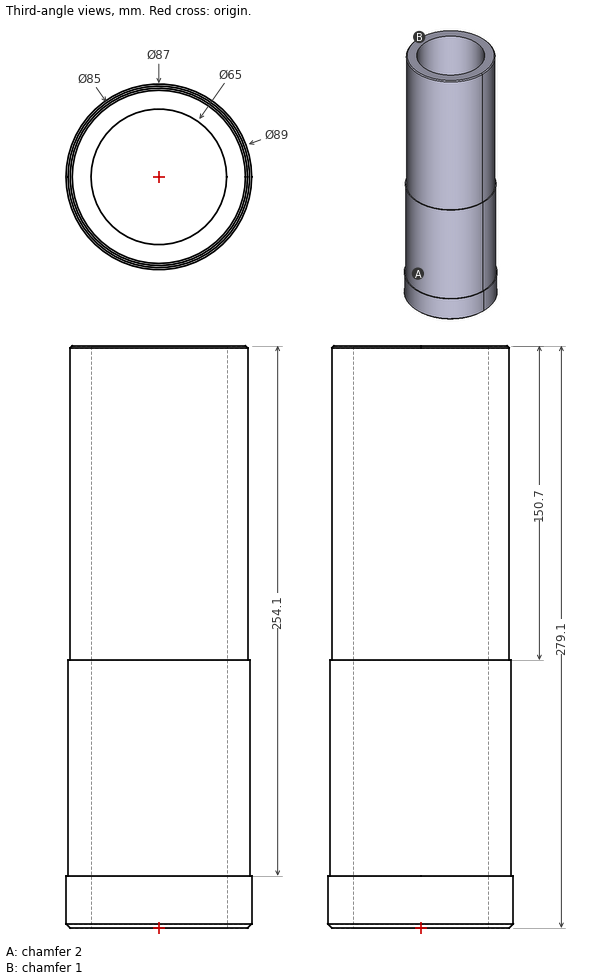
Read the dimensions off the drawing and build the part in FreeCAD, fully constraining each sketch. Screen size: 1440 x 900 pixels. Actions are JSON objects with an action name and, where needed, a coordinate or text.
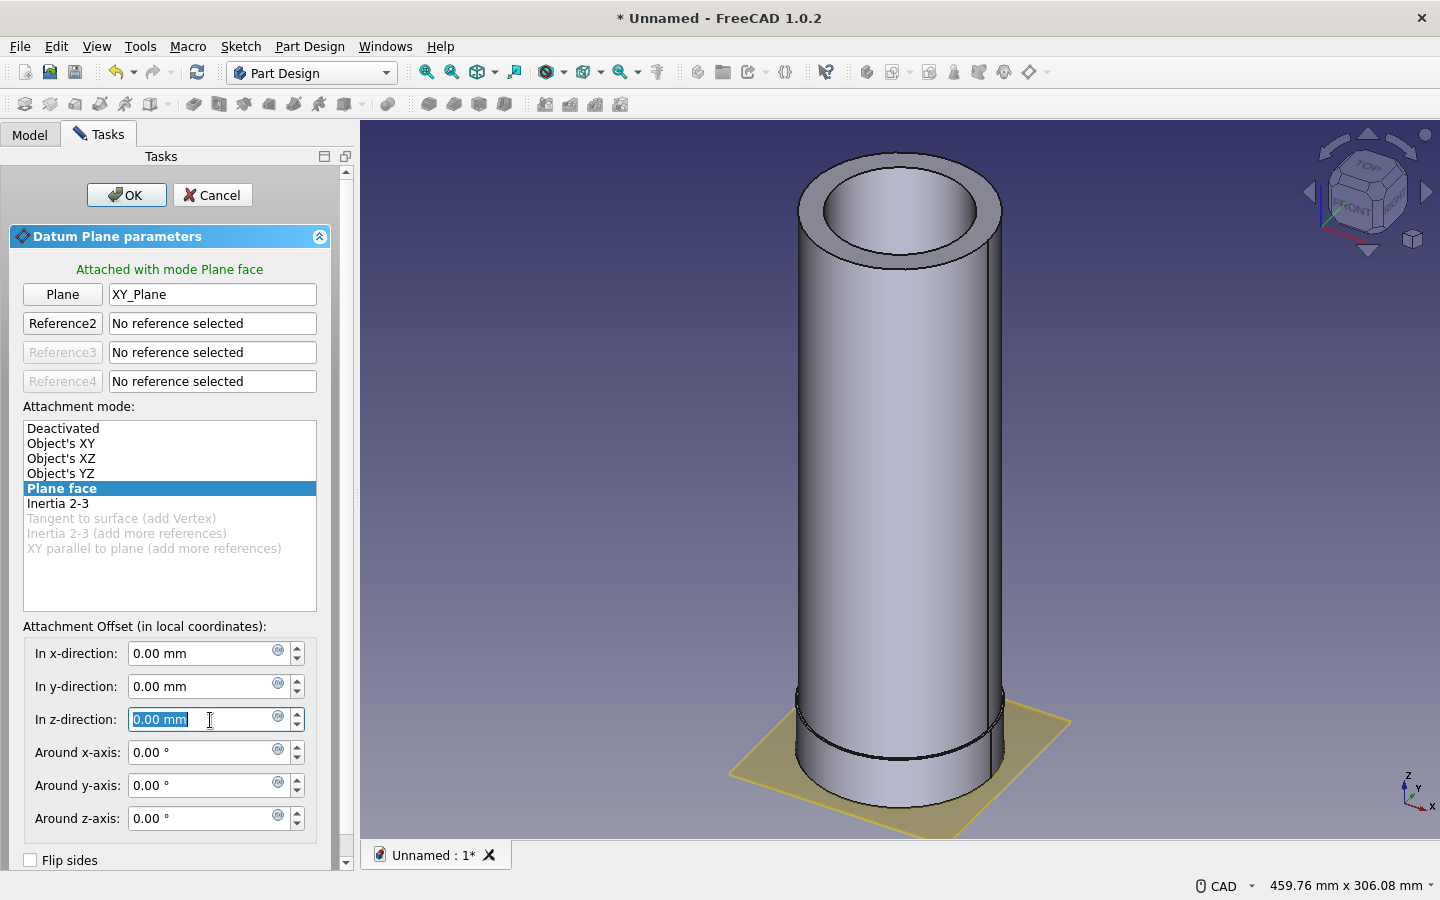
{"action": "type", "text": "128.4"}
{"action": "key", "text": "Tab"}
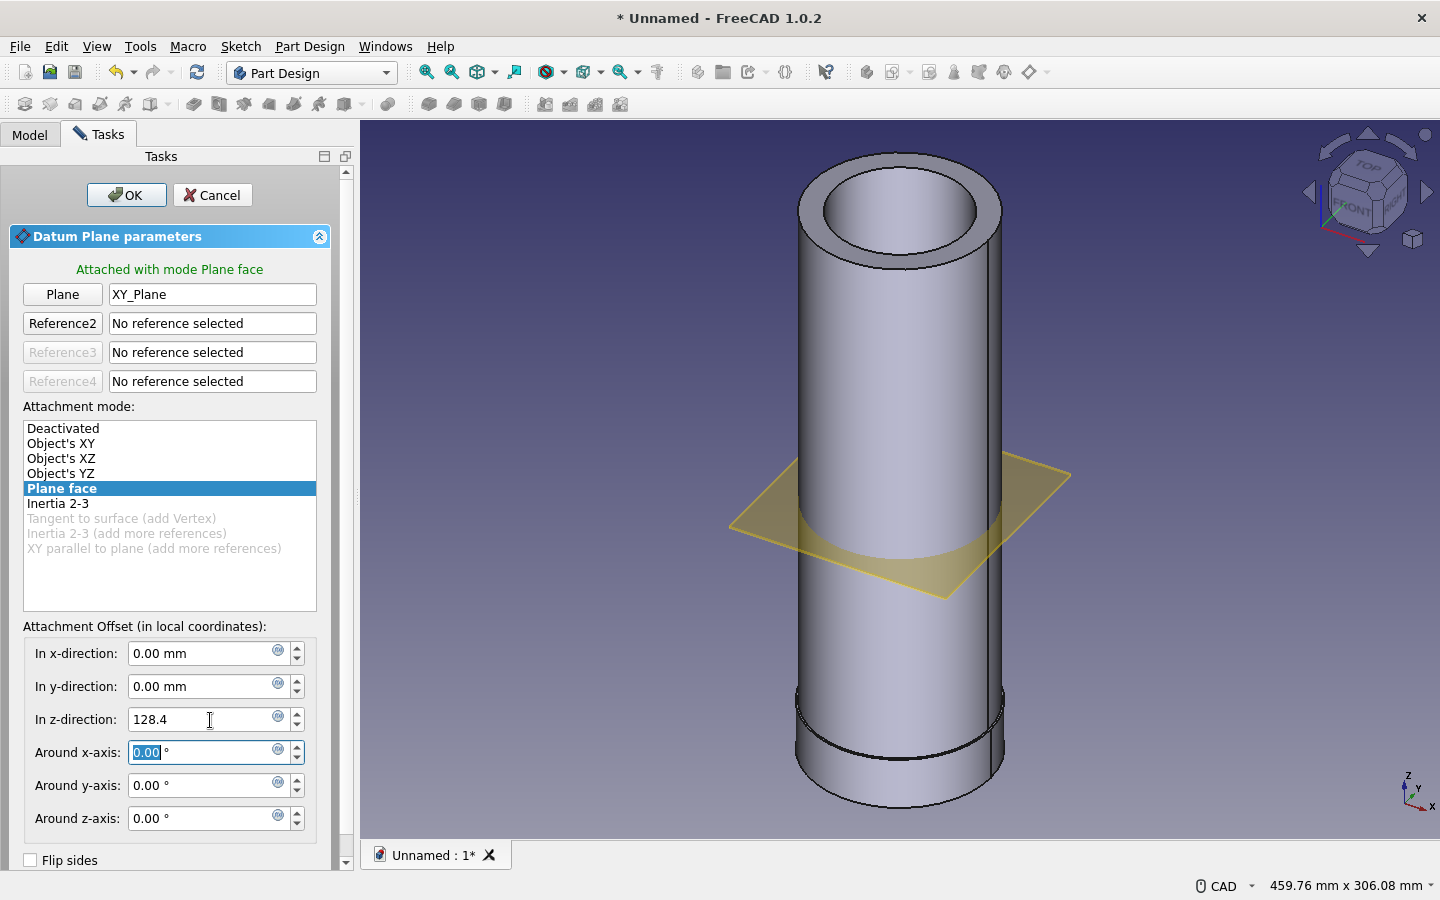
{"action": "left_click", "coordinate": [127, 195]}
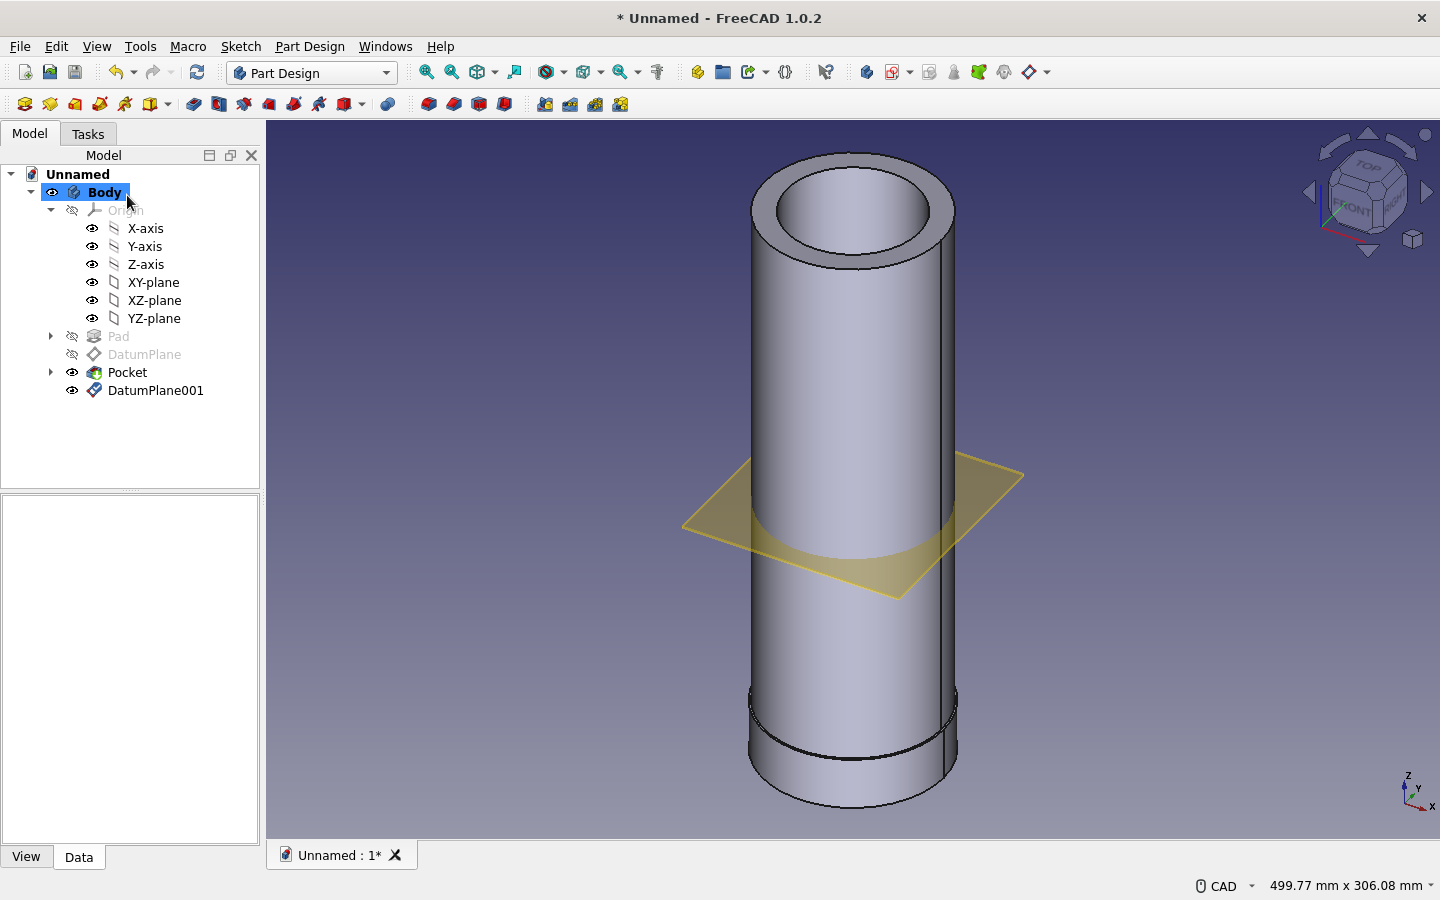
{"action": "left_click", "coordinate": [117, 390]}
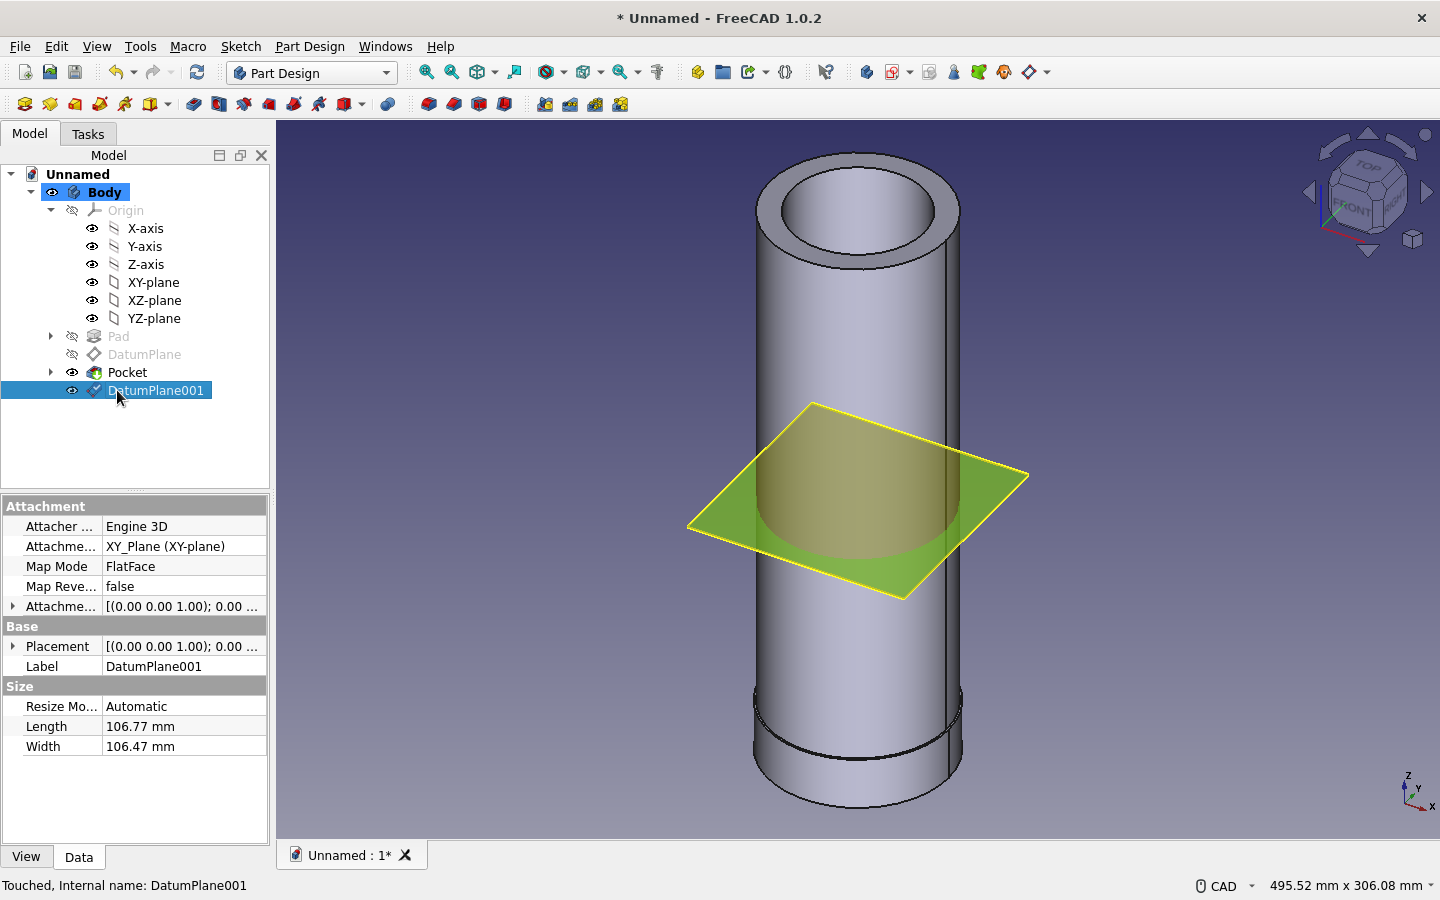
{"action": "left_click", "coordinate": [892, 72]}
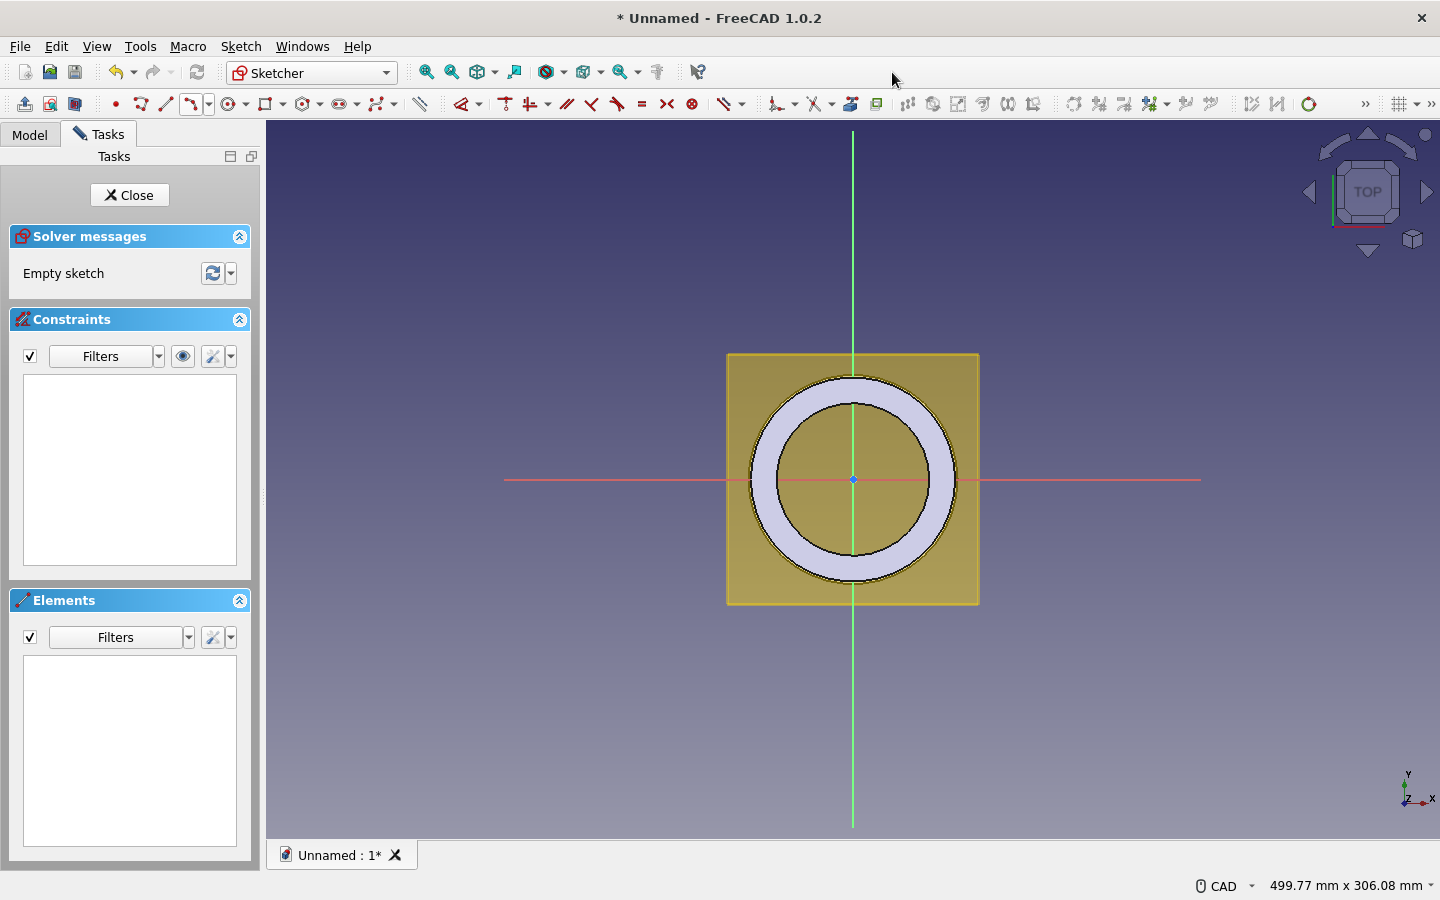
{"action": "left_click", "coordinate": [75, 104]}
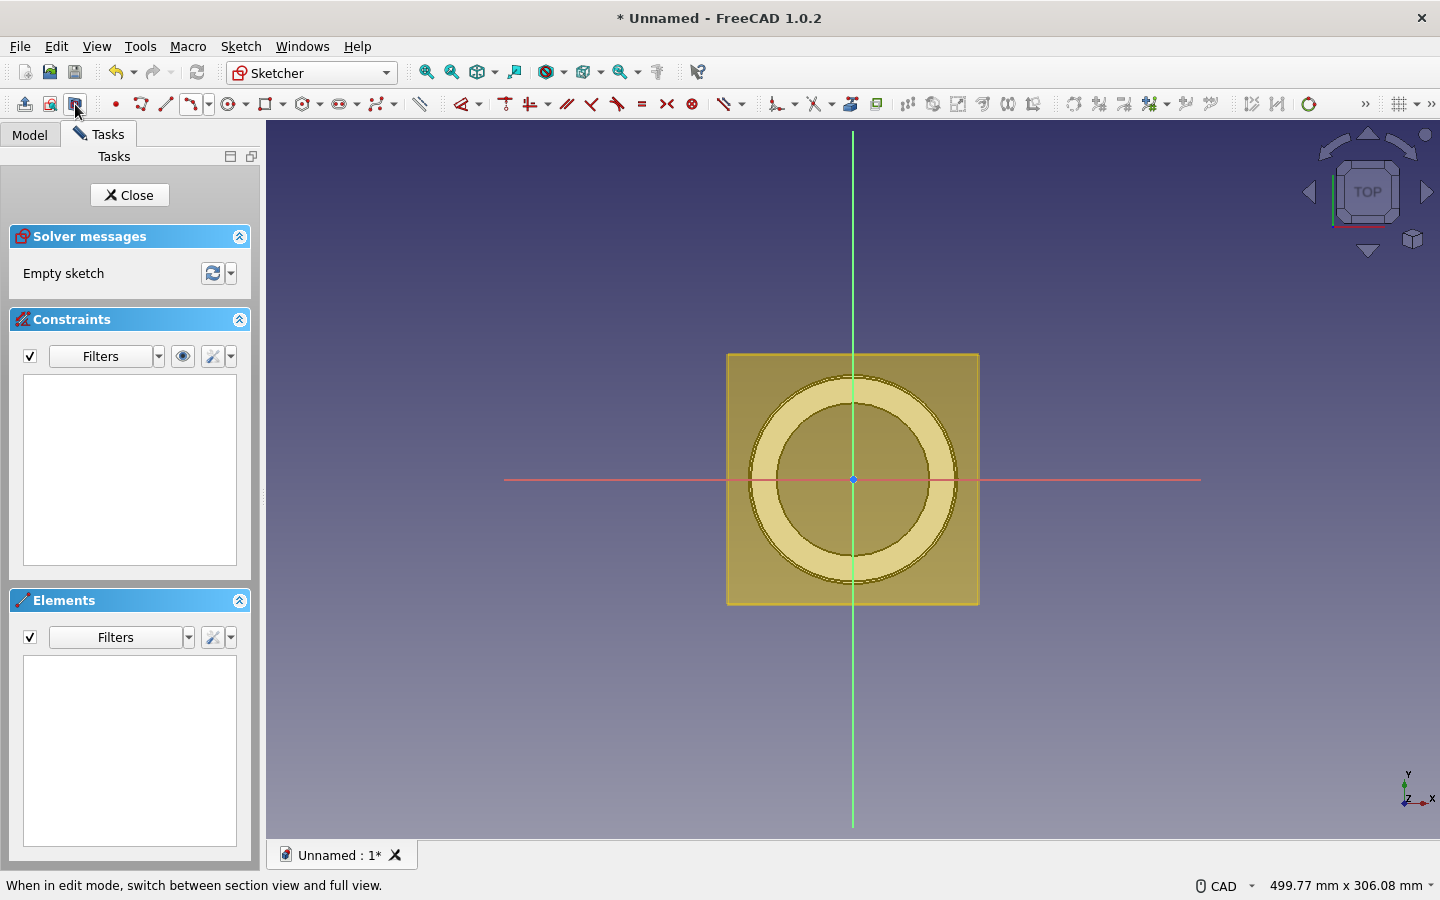
{"action": "scroll", "coordinate": [909, 480], "scroll_direction": "up", "scroll_amount": 4}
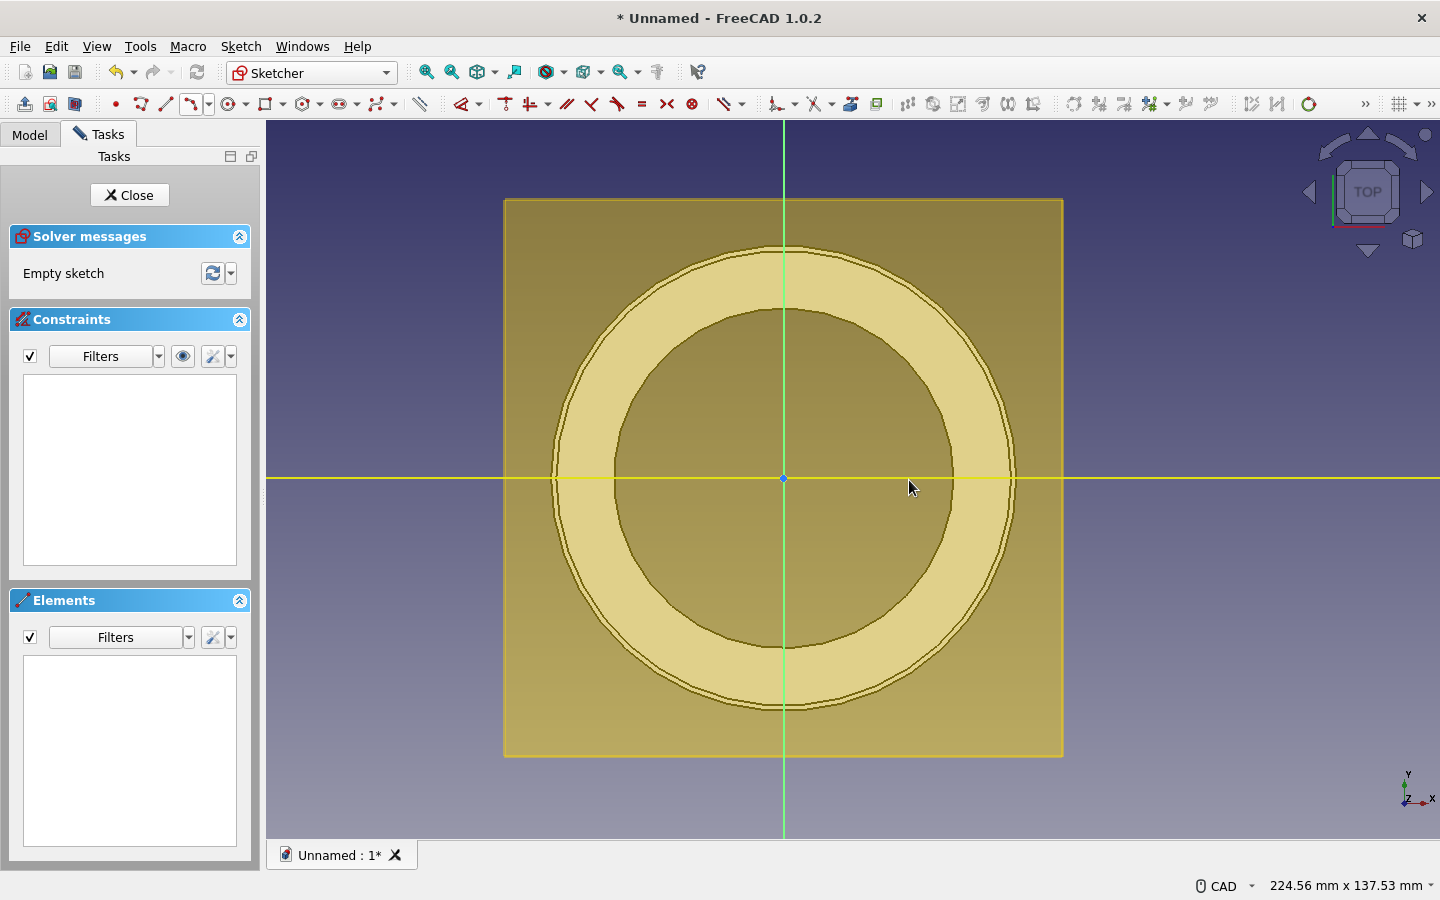
{"action": "left_click", "coordinate": [228, 104]}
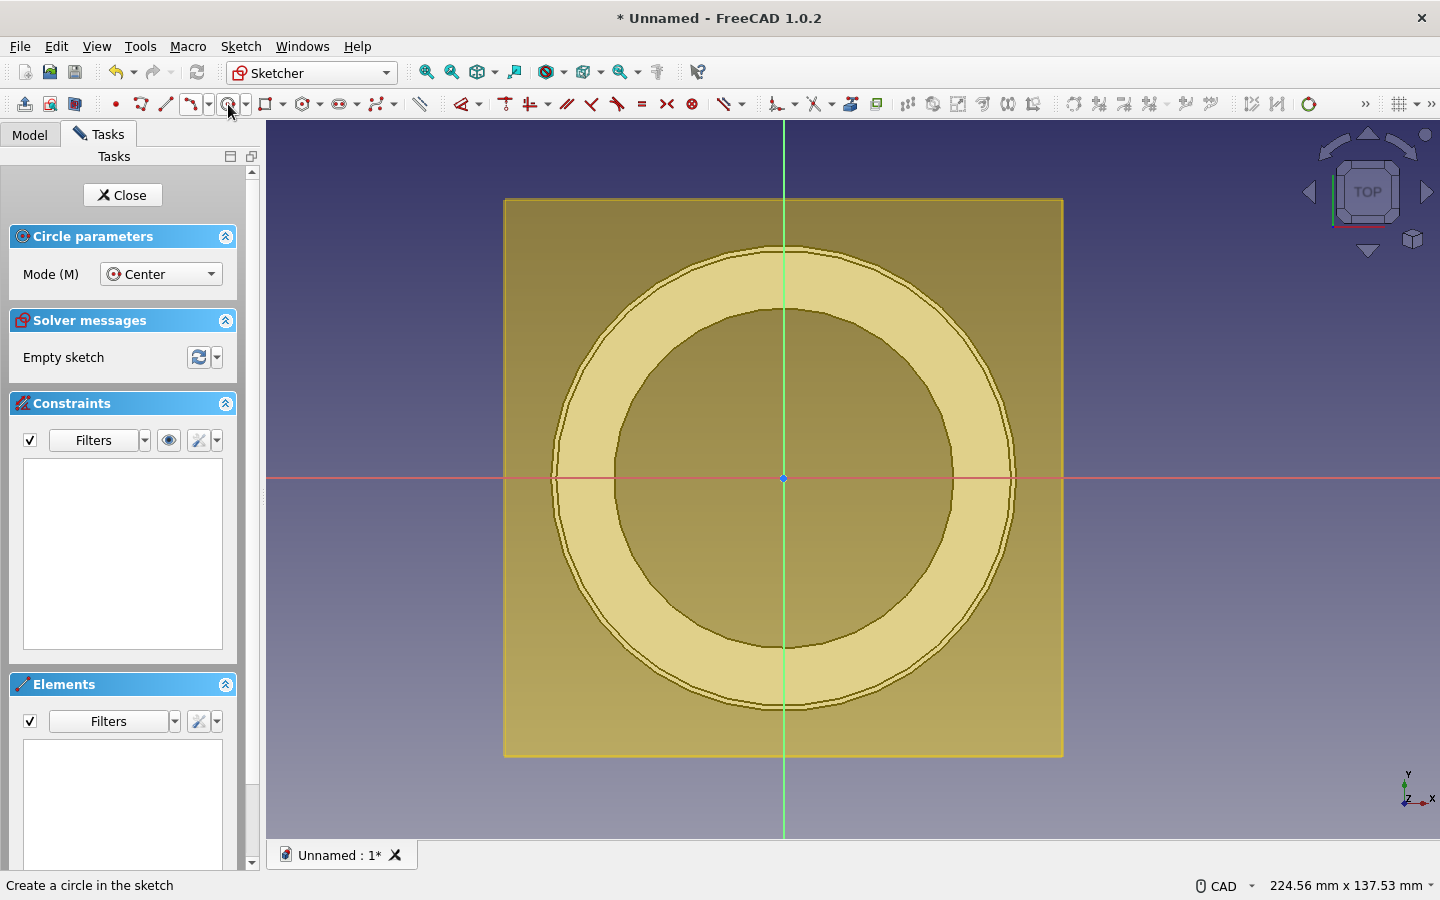
{"action": "left_click", "coordinate": [784, 478]}
{"action": "mouse_move", "coordinate": [945, 317]}